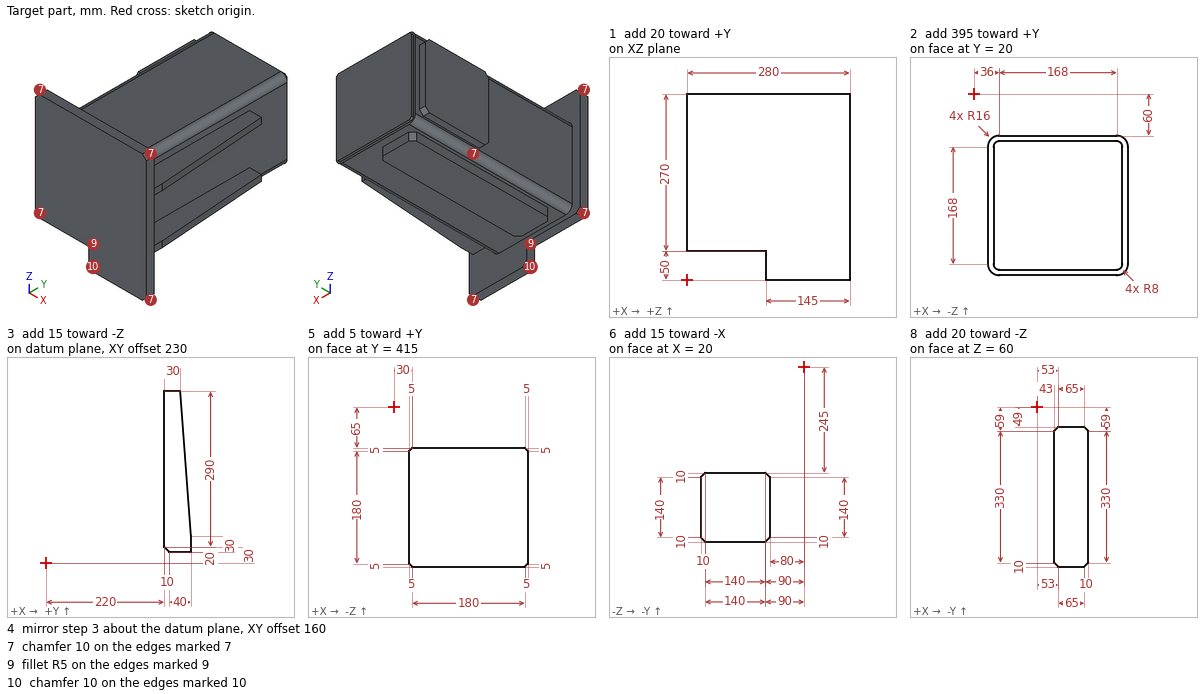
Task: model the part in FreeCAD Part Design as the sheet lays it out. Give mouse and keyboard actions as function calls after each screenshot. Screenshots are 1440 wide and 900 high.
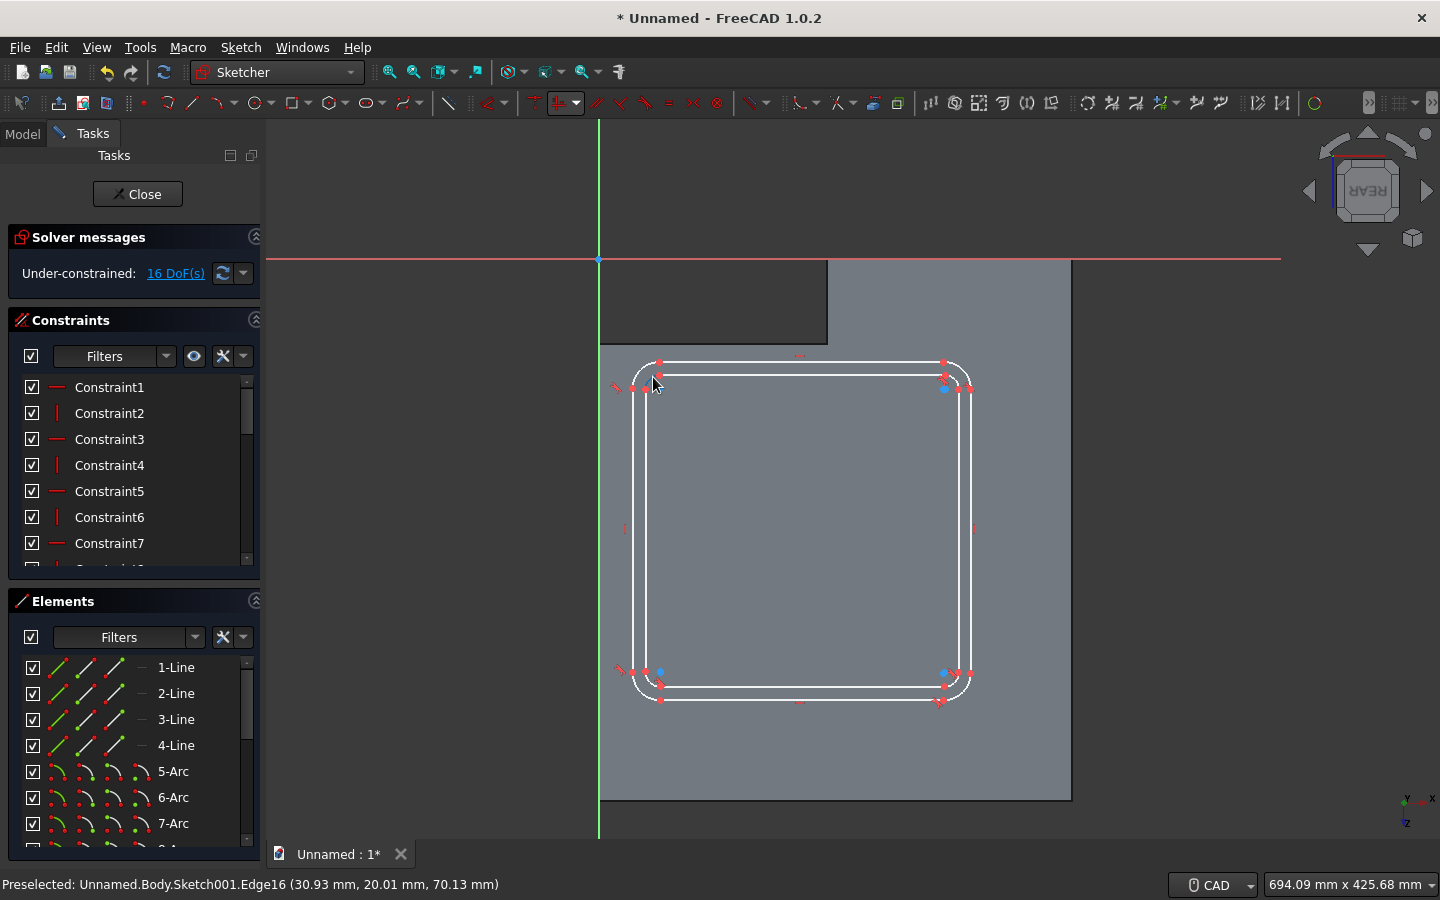
click(968, 377)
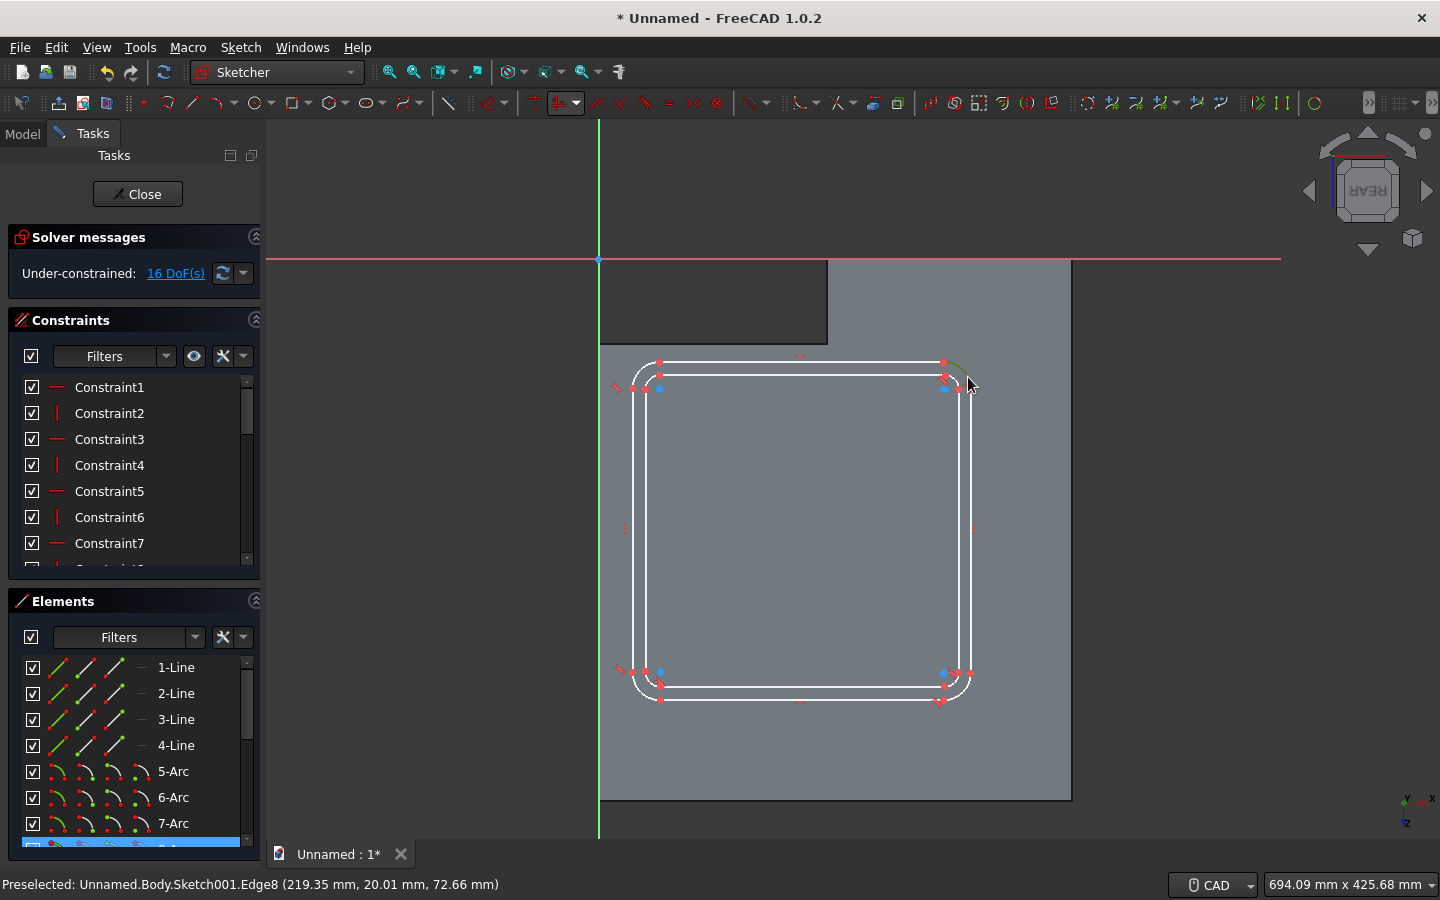
scroll(955, 379, up, 2)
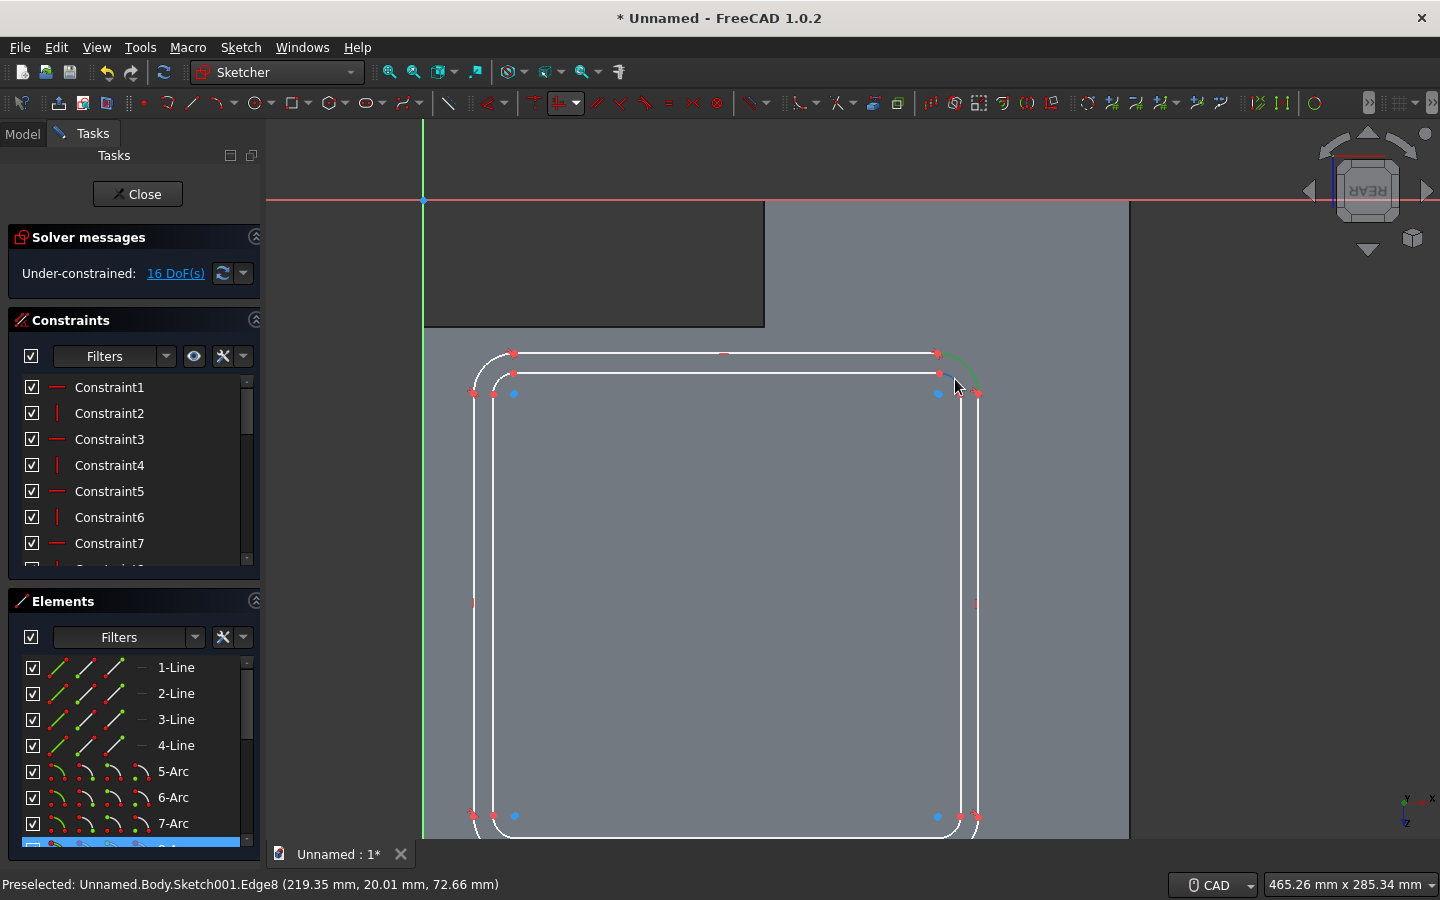
click(955, 380)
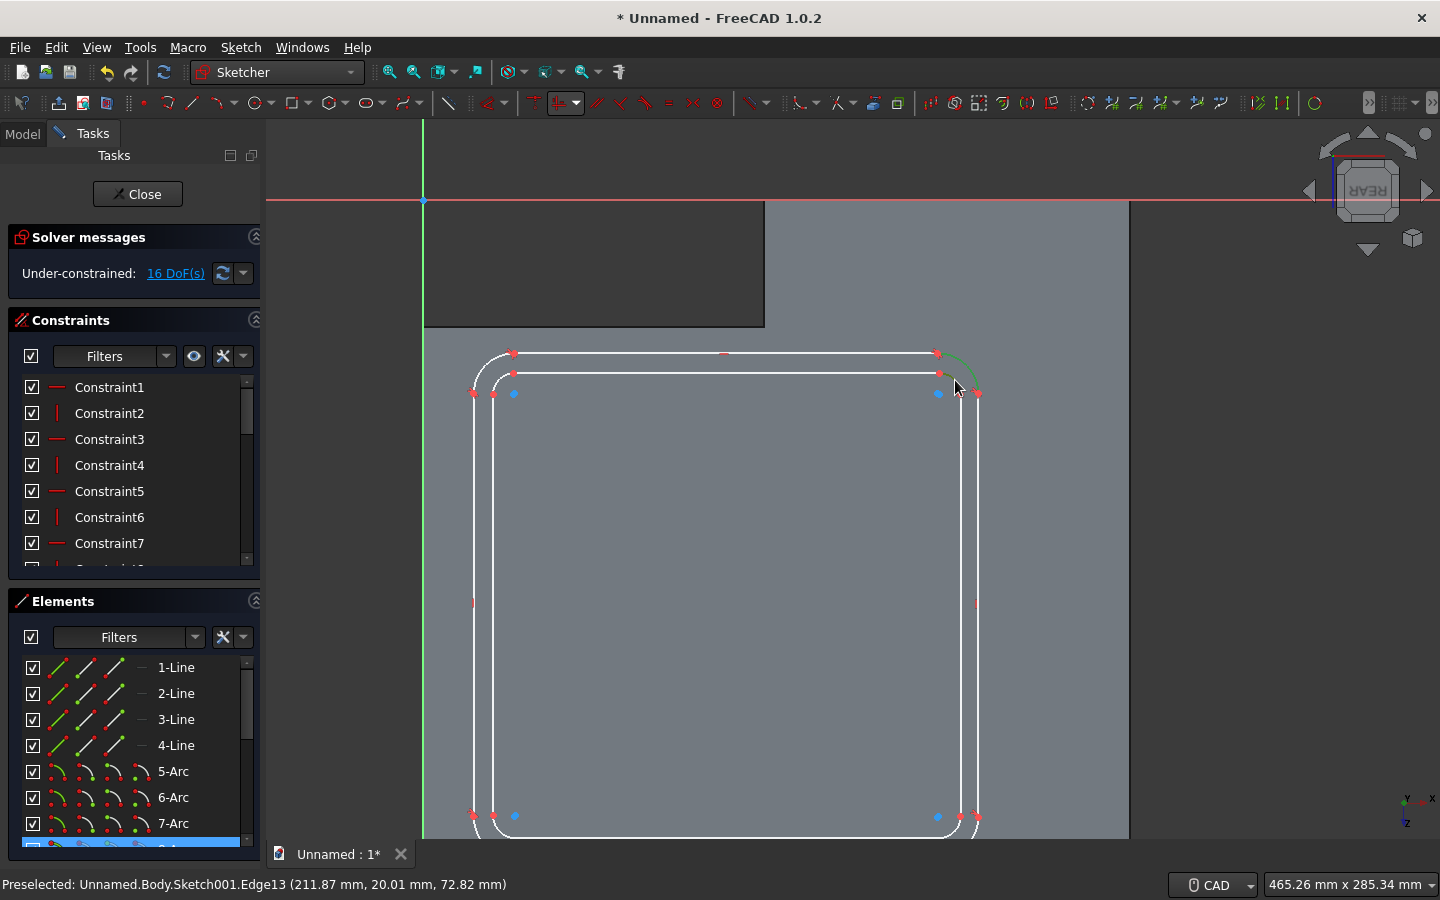
click(534, 104)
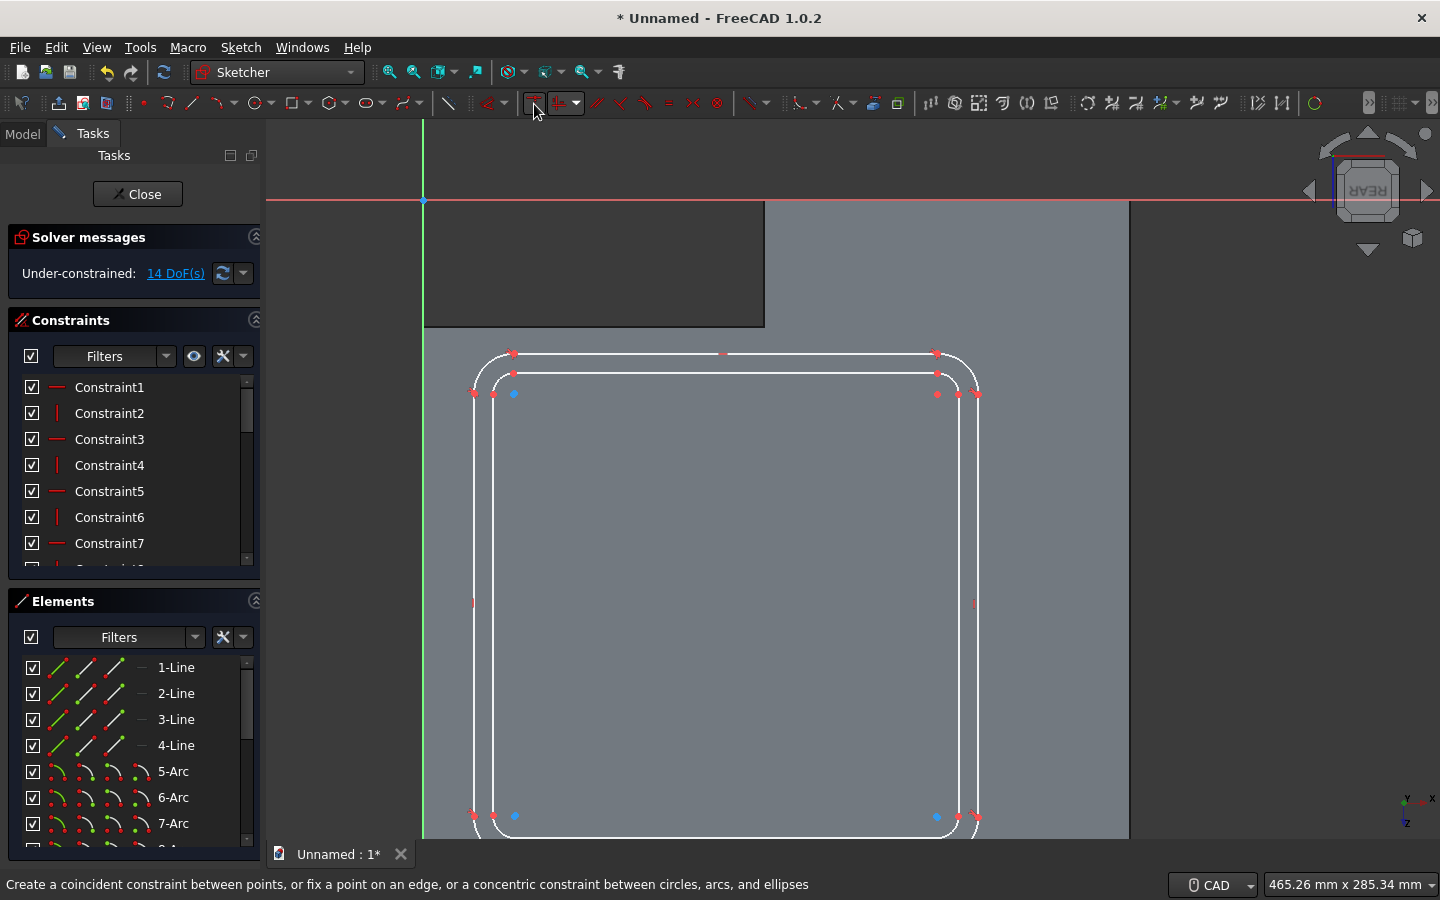
scroll(954, 378, down, 2)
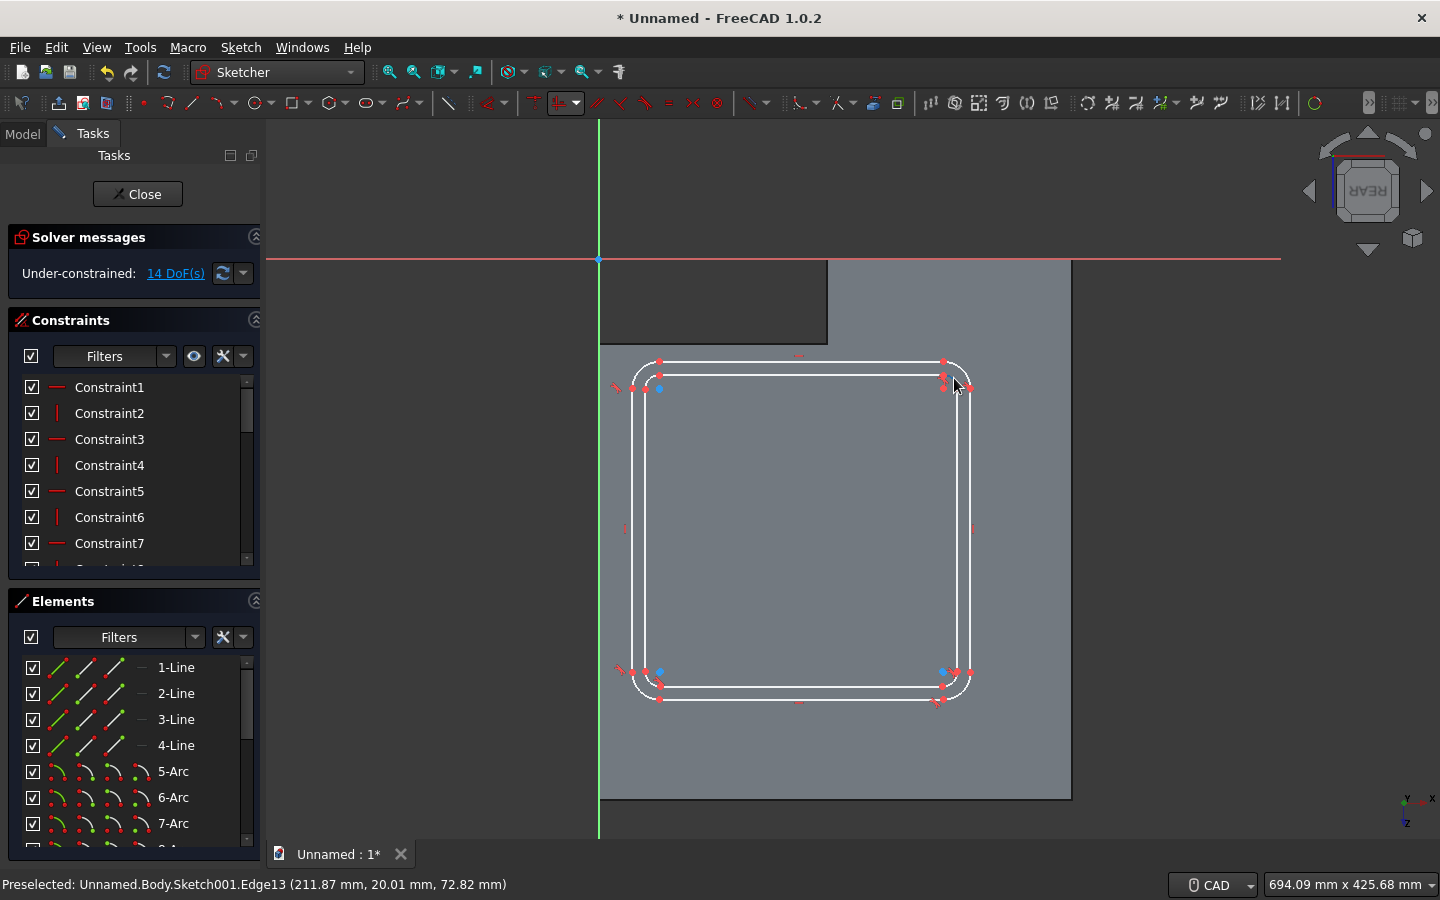
click(956, 697)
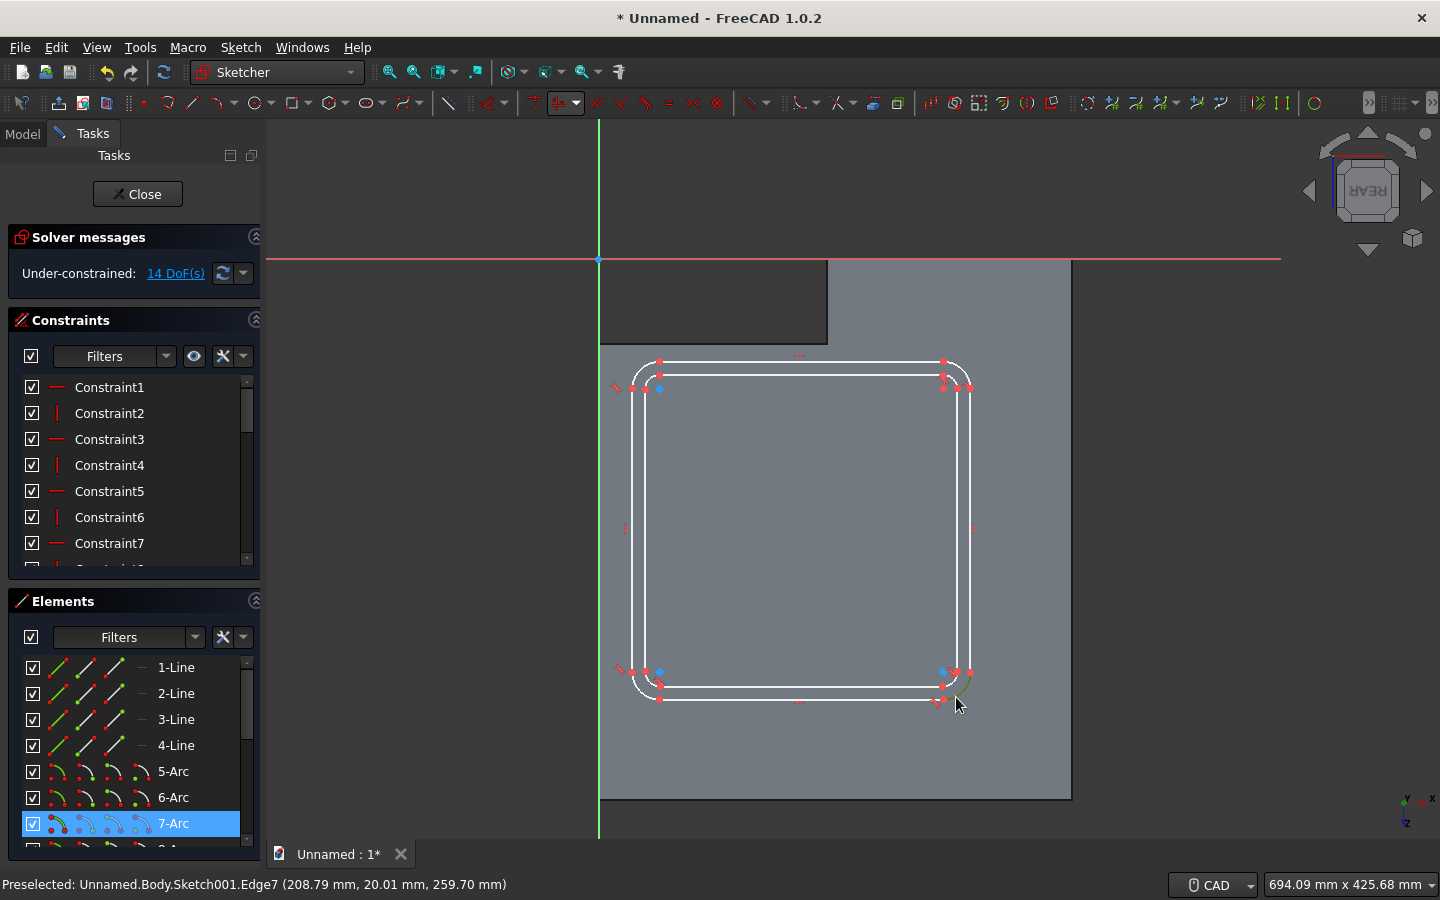
scroll(953, 682, up, 2)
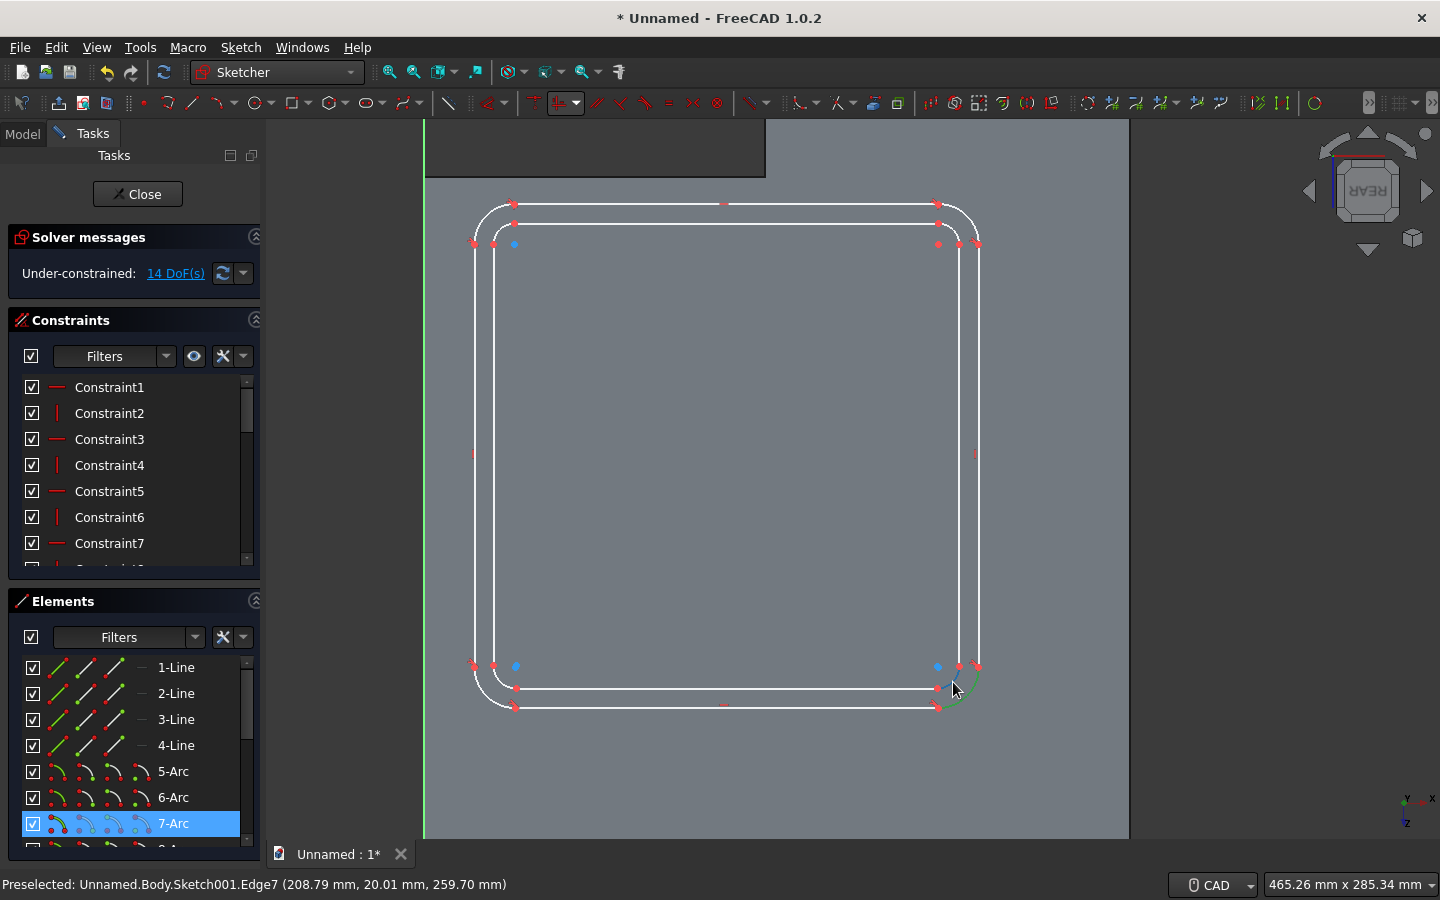
click(953, 682)